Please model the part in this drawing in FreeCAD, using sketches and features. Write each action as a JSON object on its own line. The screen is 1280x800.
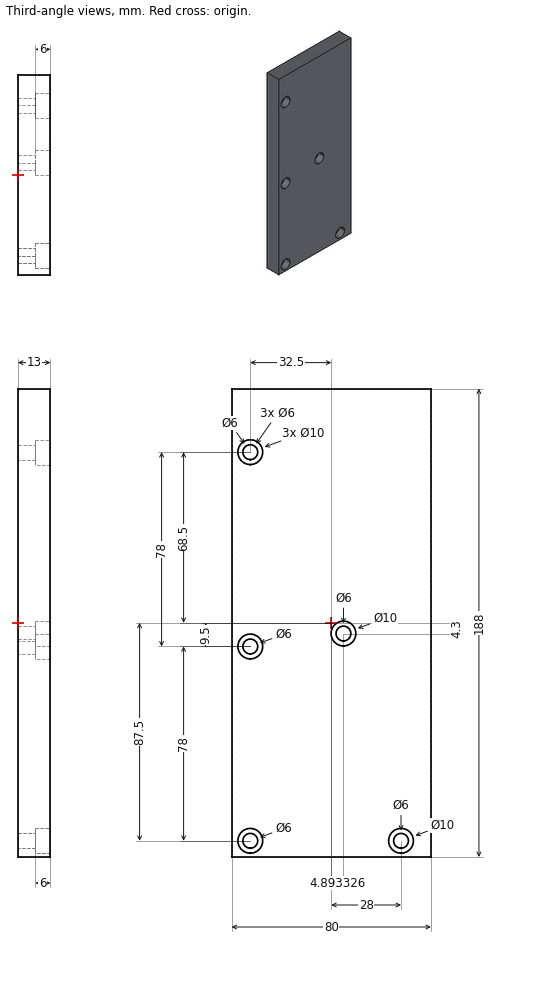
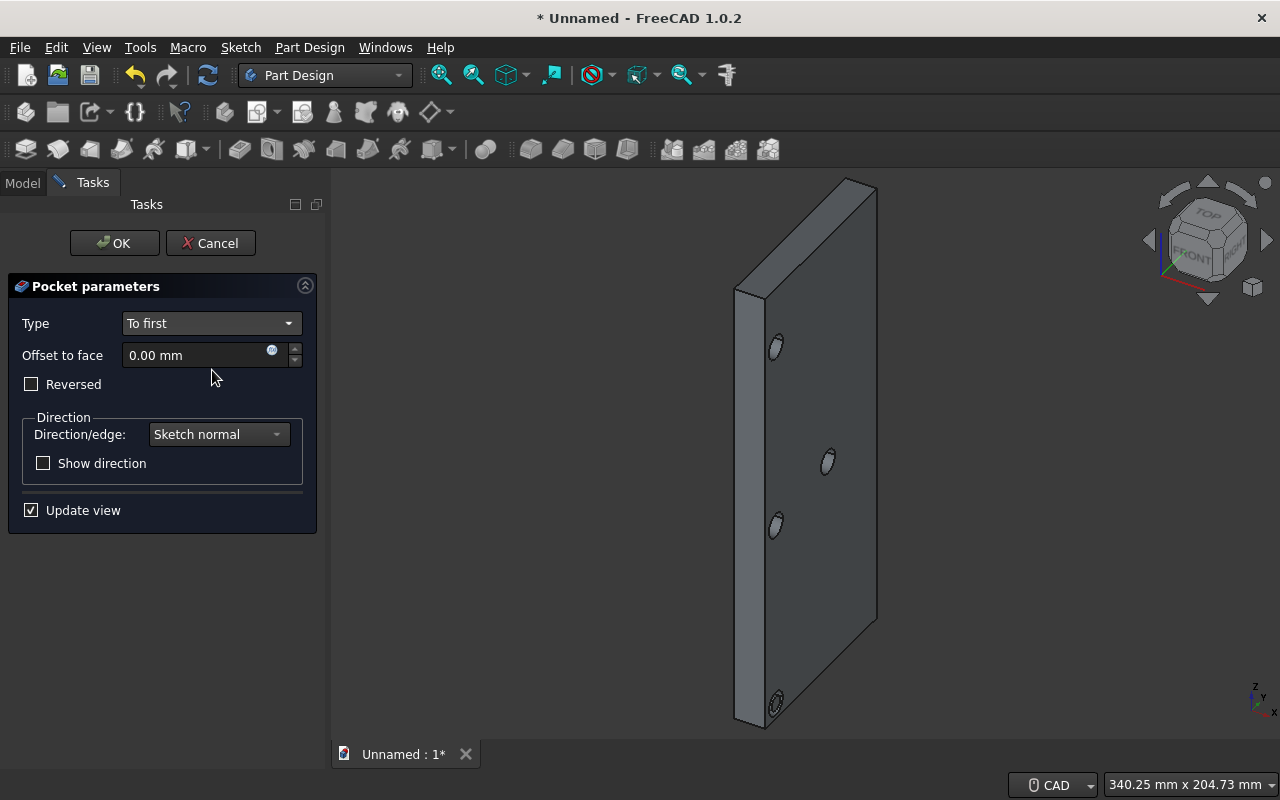
{"action": "left_click", "coordinate": [115, 243]}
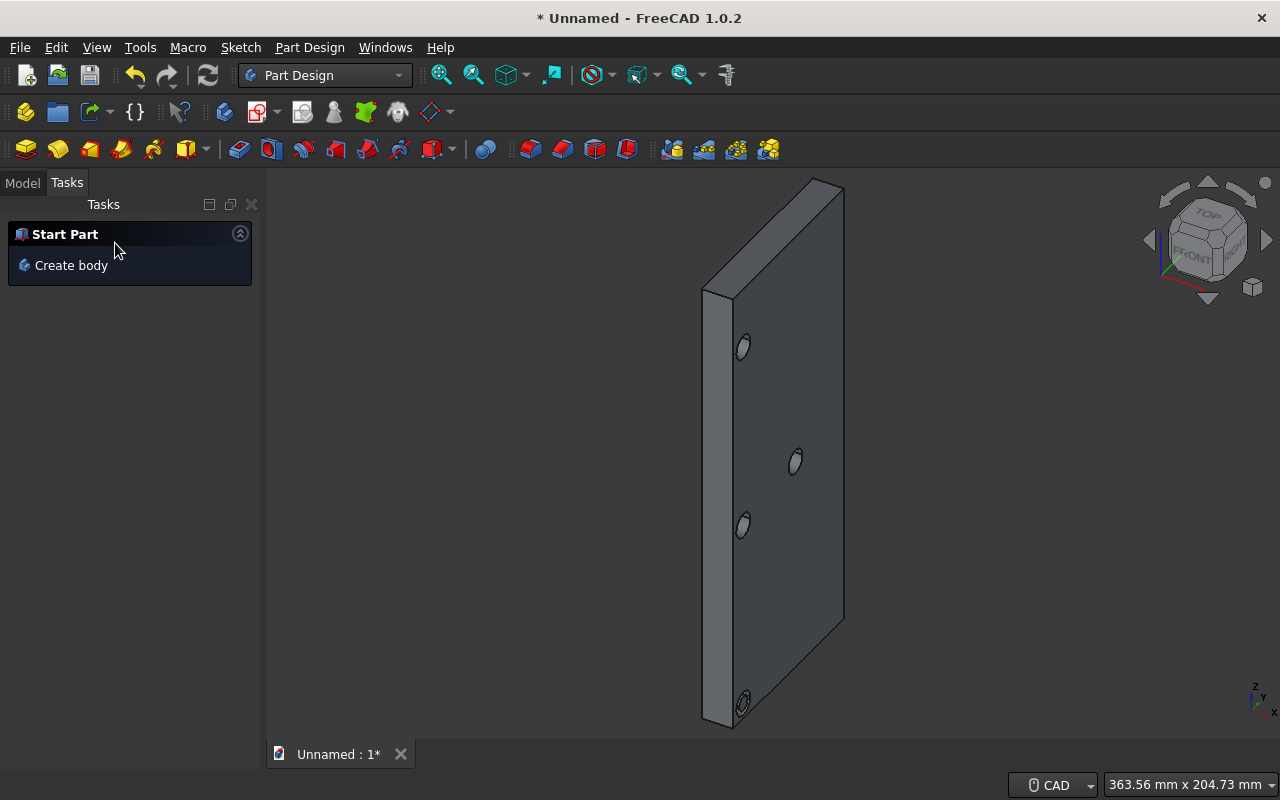
{"action": "left_click", "coordinate": [789, 580]}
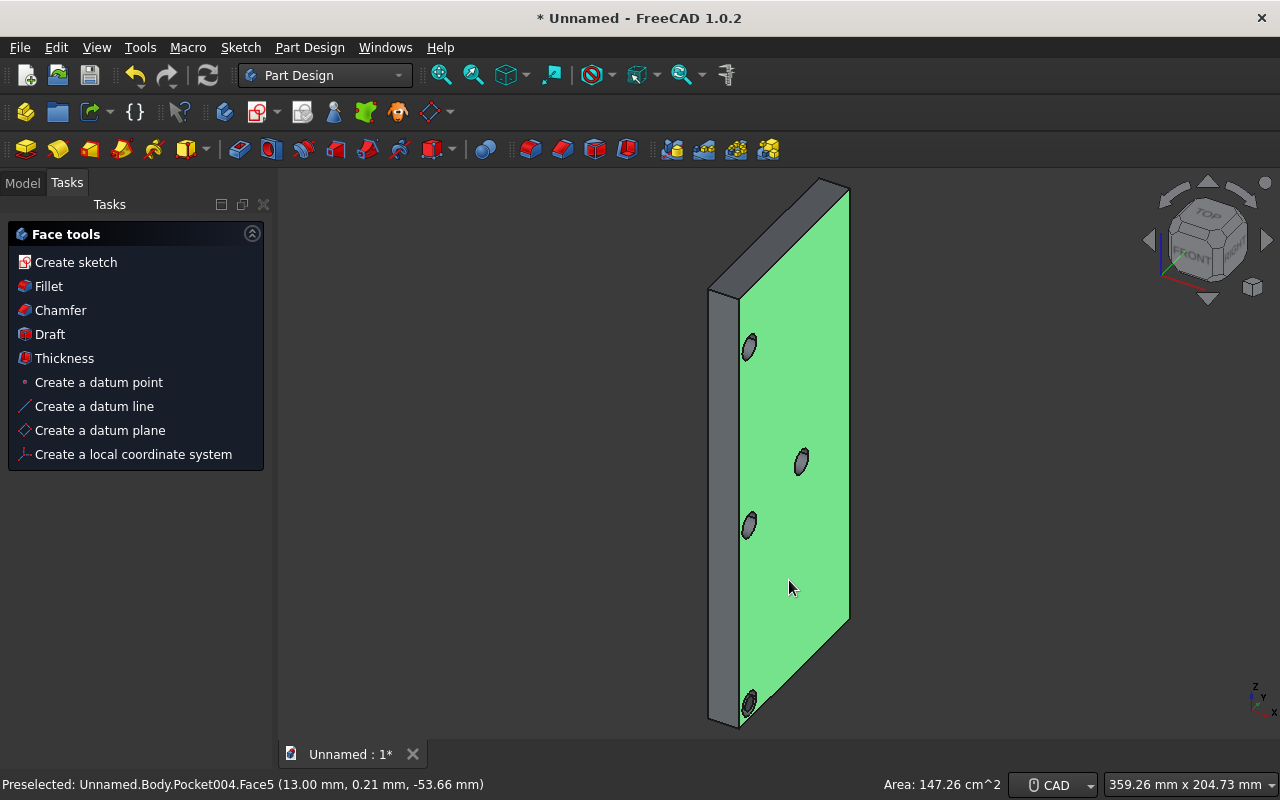
{"action": "left_click", "coordinate": [258, 112]}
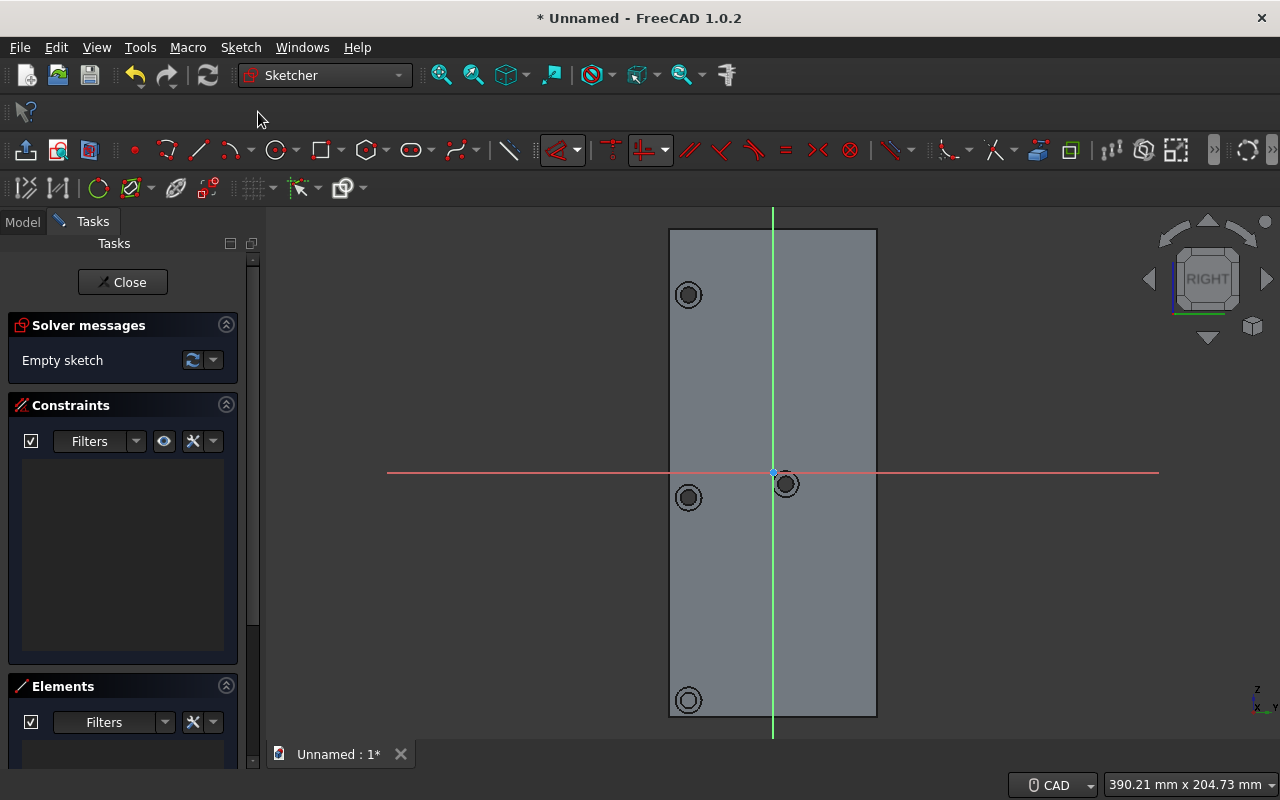
{"action": "scroll", "coordinate": [688, 711], "scroll_direction": "up", "scroll_amount": 15}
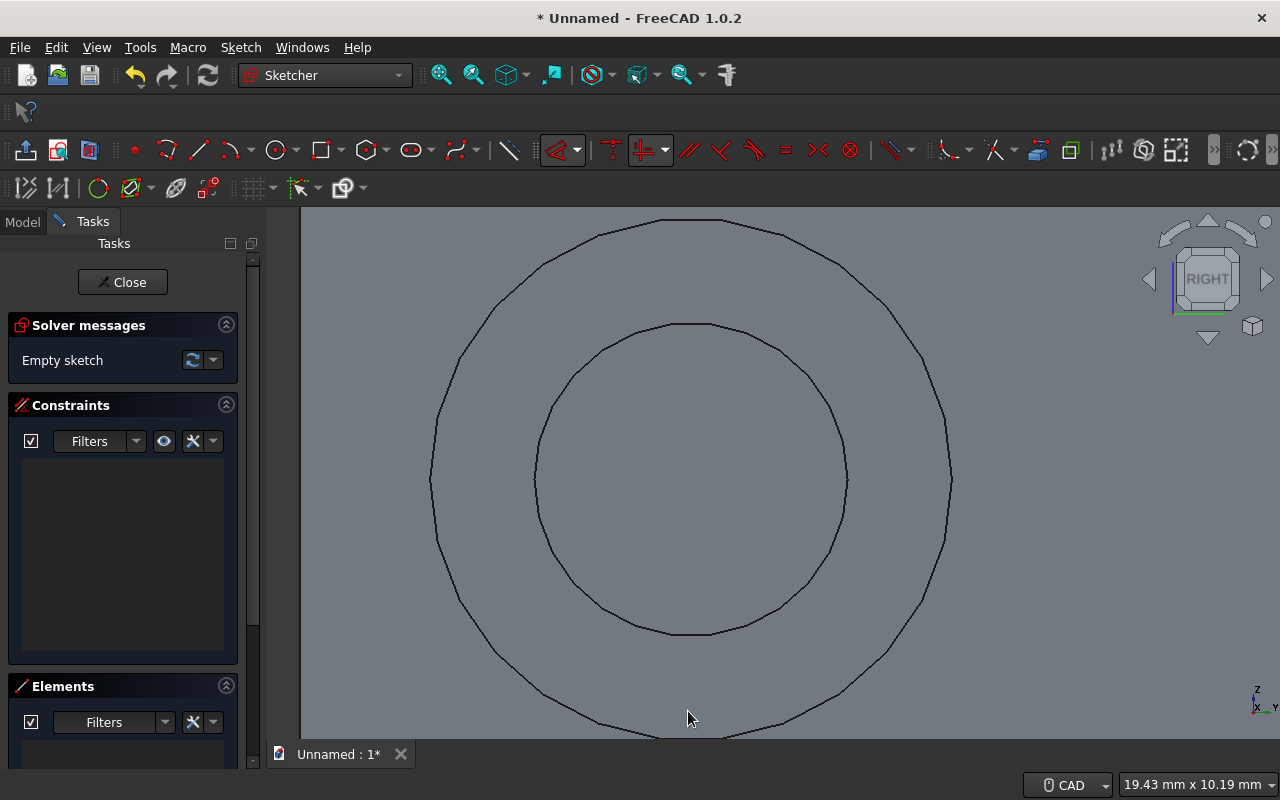
{"action": "left_click", "coordinate": [276, 150]}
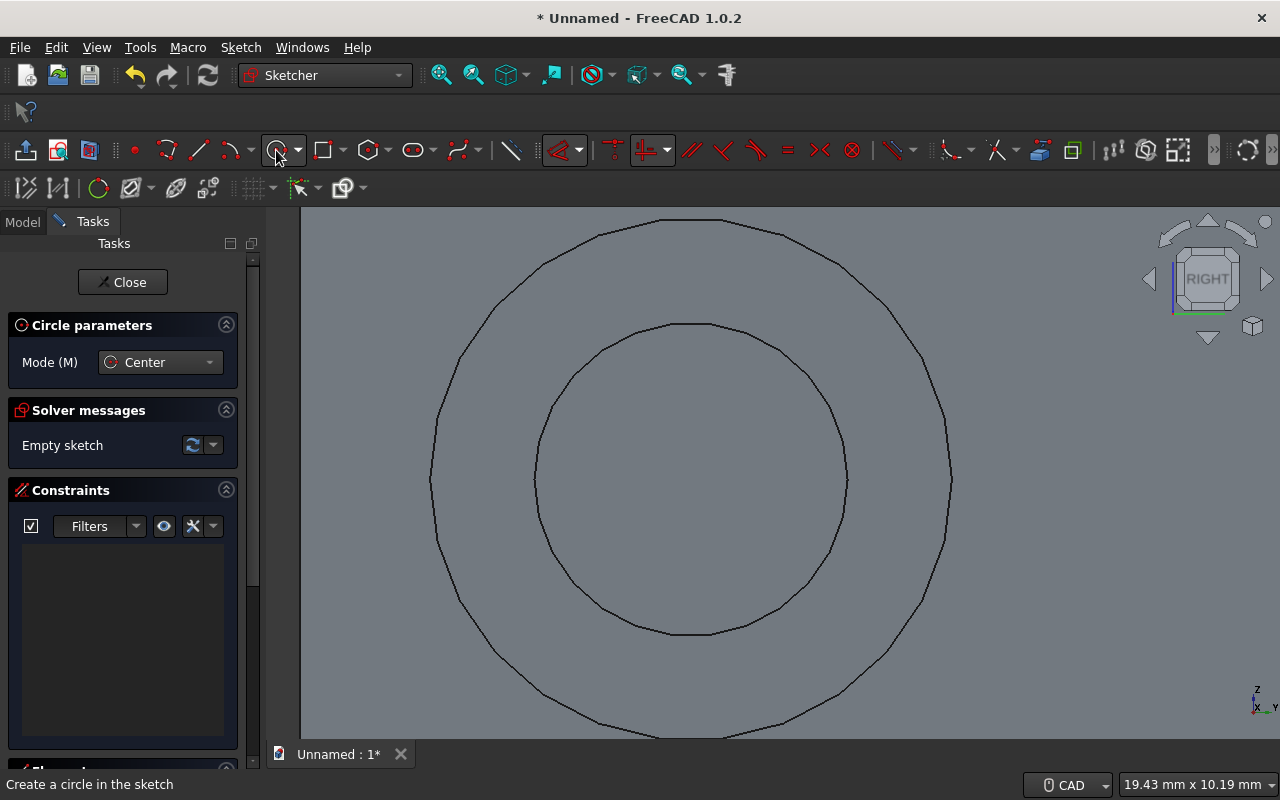
{"action": "left_click", "coordinate": [691, 480]}
{"action": "left_click", "coordinate": [802, 369]}
{"action": "key", "text": "Escape"}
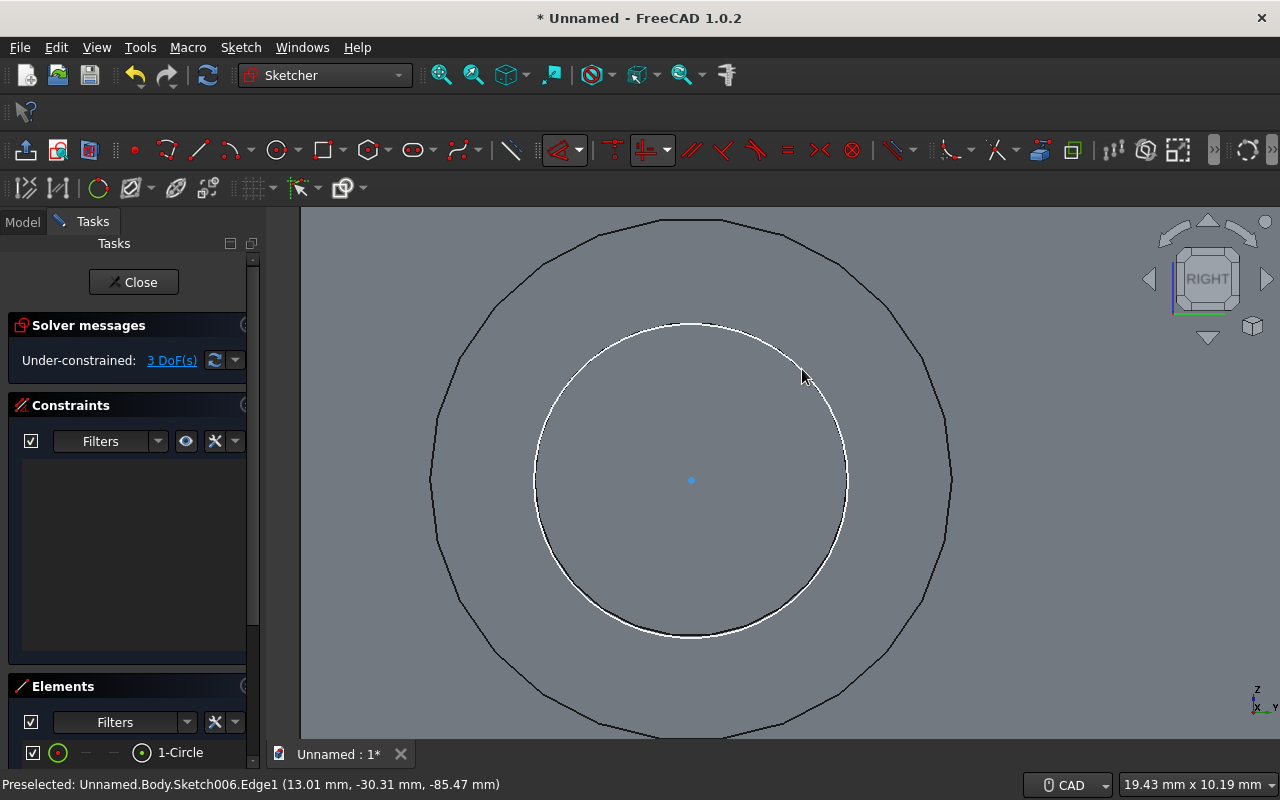
{"action": "left_click", "coordinate": [802, 370]}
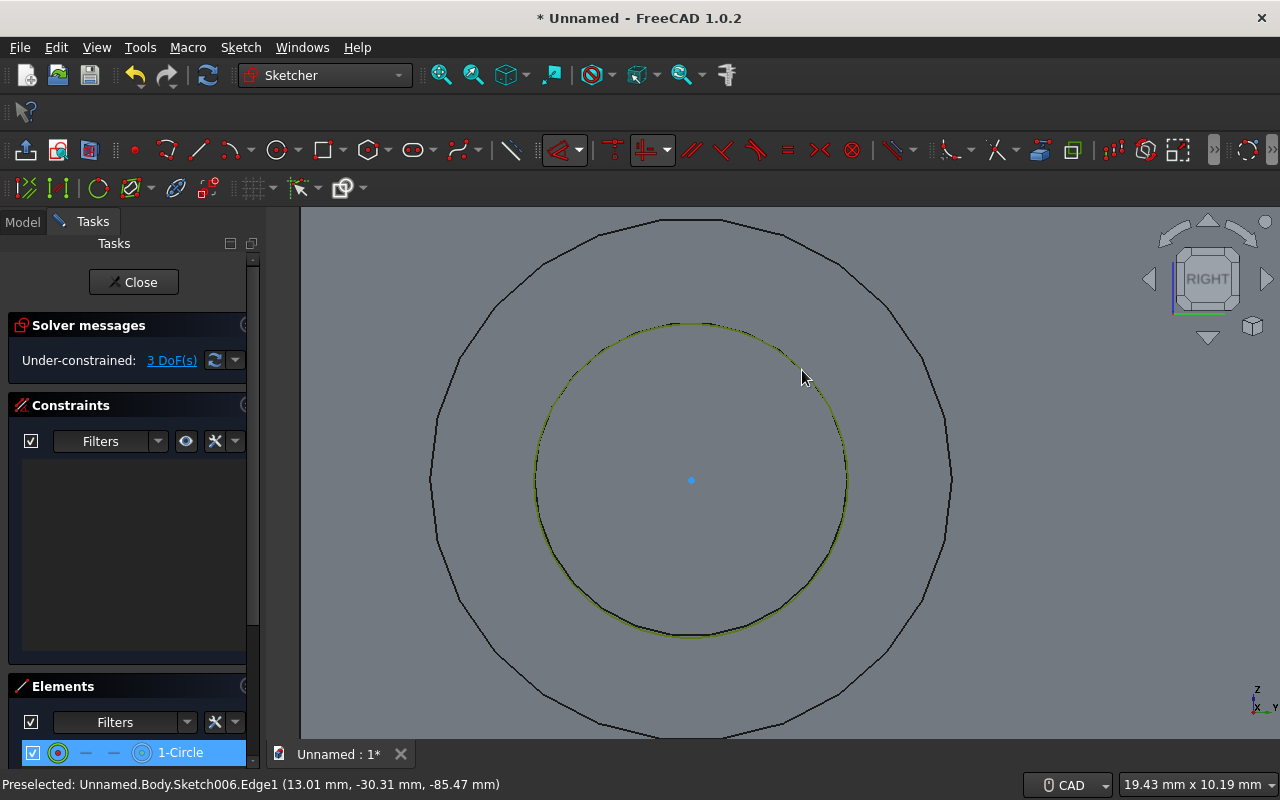
{"action": "key", "text": "k o"}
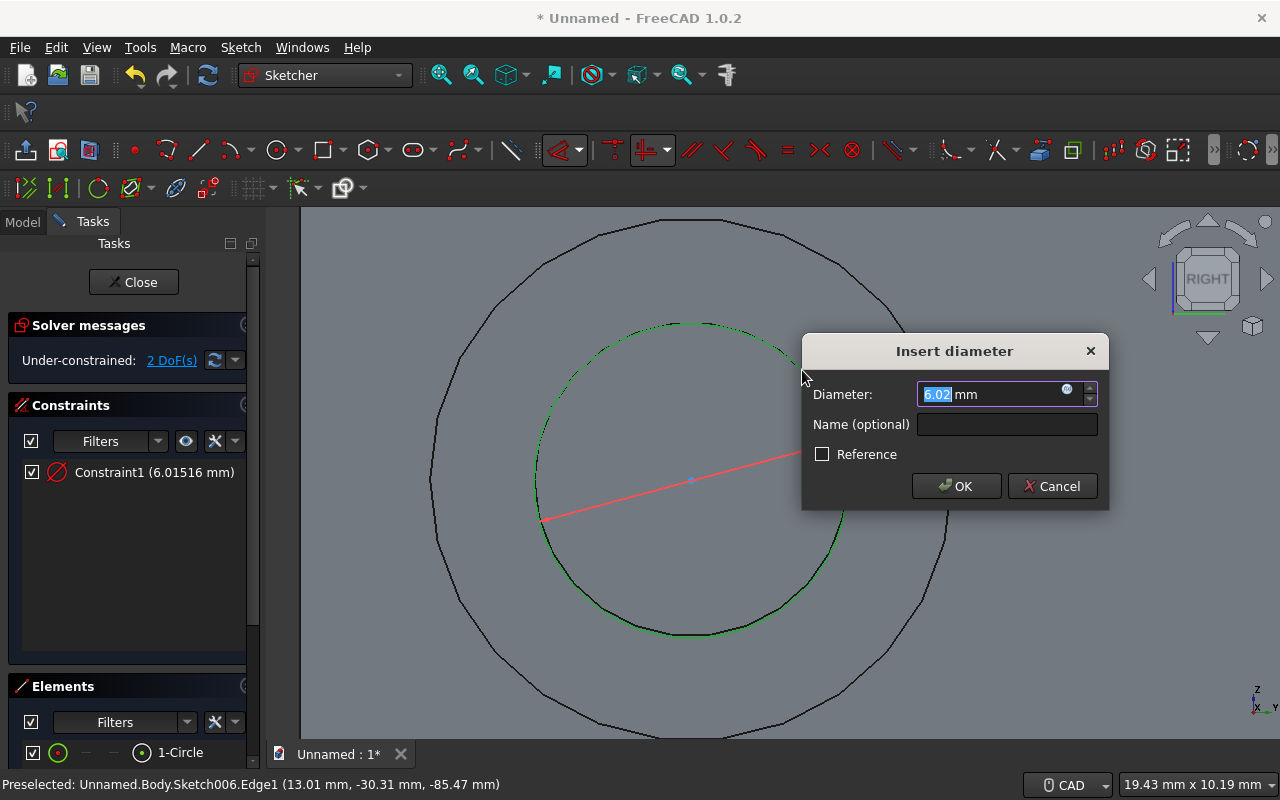
{"action": "type", "text": "6"}
{"action": "key", "text": "Return"}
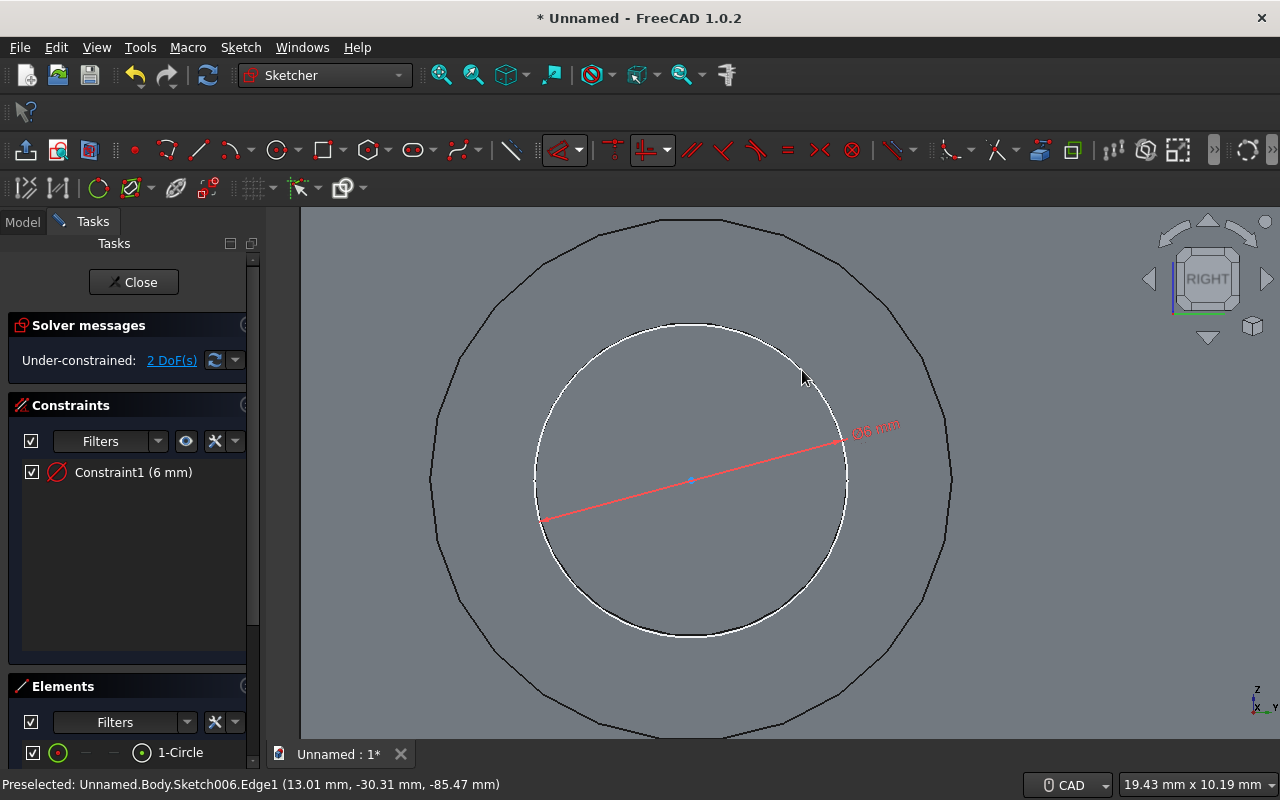
{"action": "left_click", "coordinate": [691, 481]}